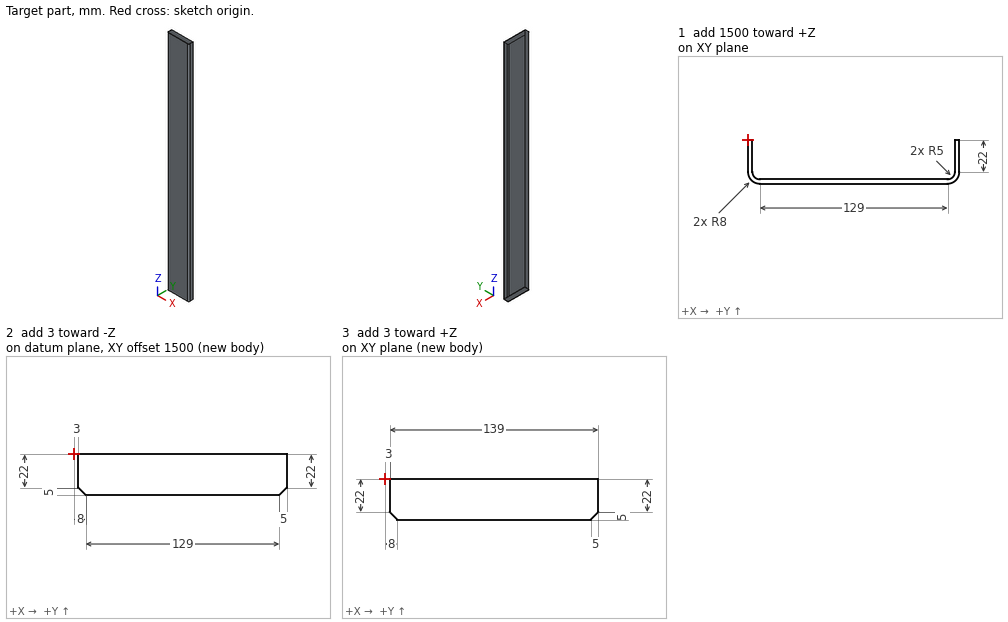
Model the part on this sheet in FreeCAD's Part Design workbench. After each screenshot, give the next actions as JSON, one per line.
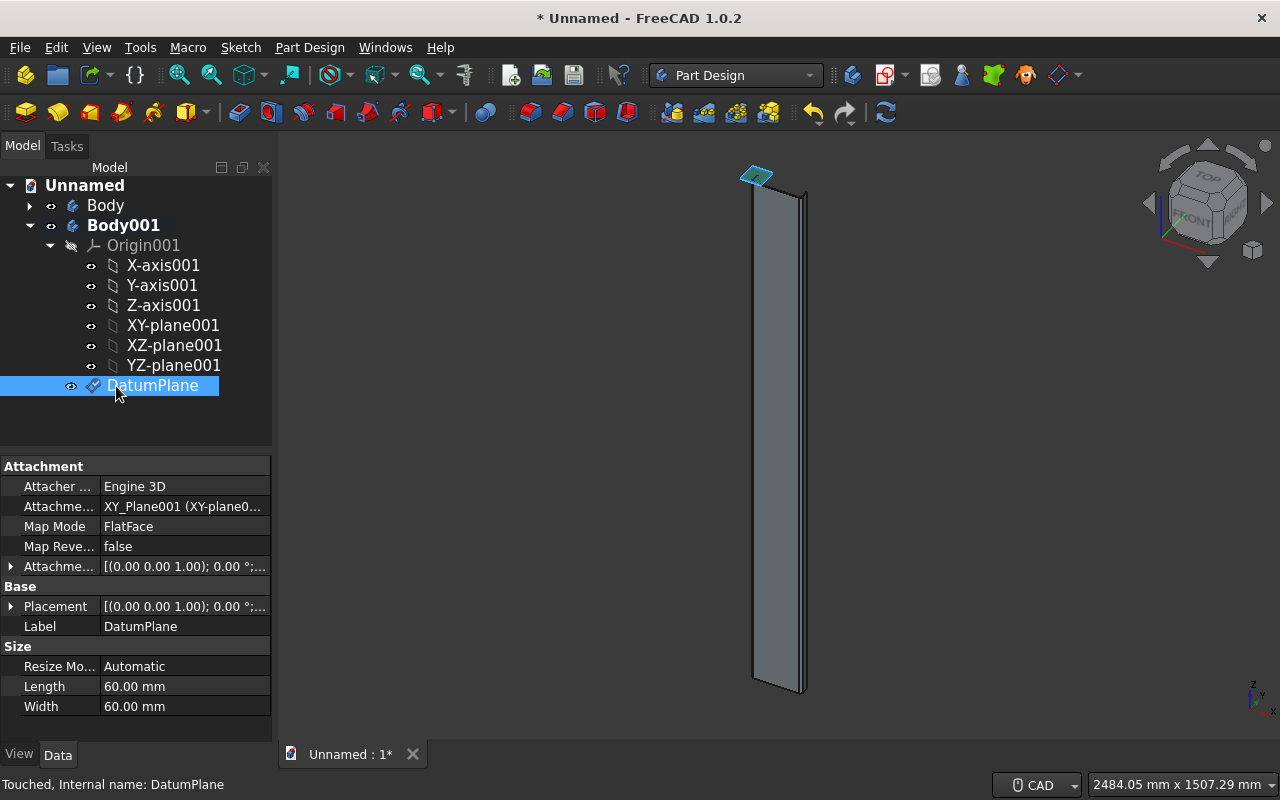
{"action": "left_click", "coordinate": [886, 76]}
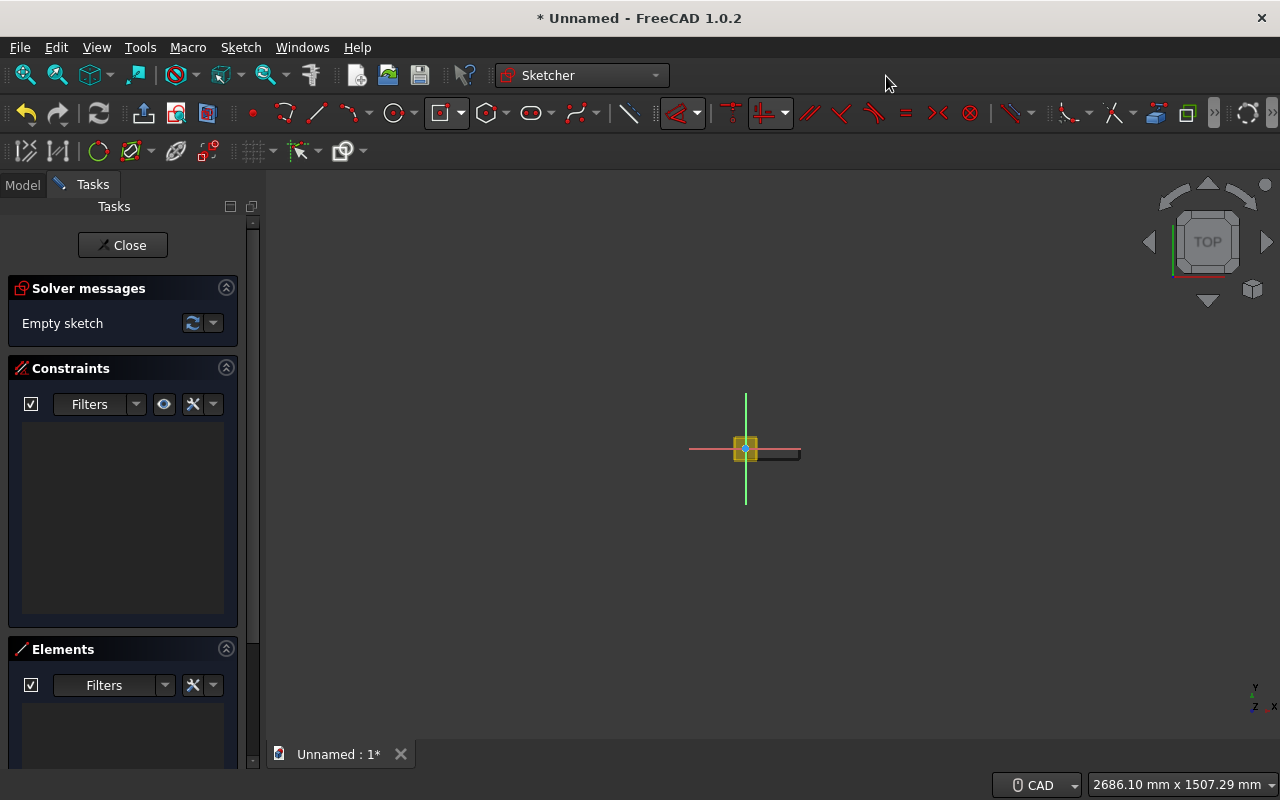
{"action": "scroll", "coordinate": [779, 454], "scroll_direction": "up", "scroll_amount": 12}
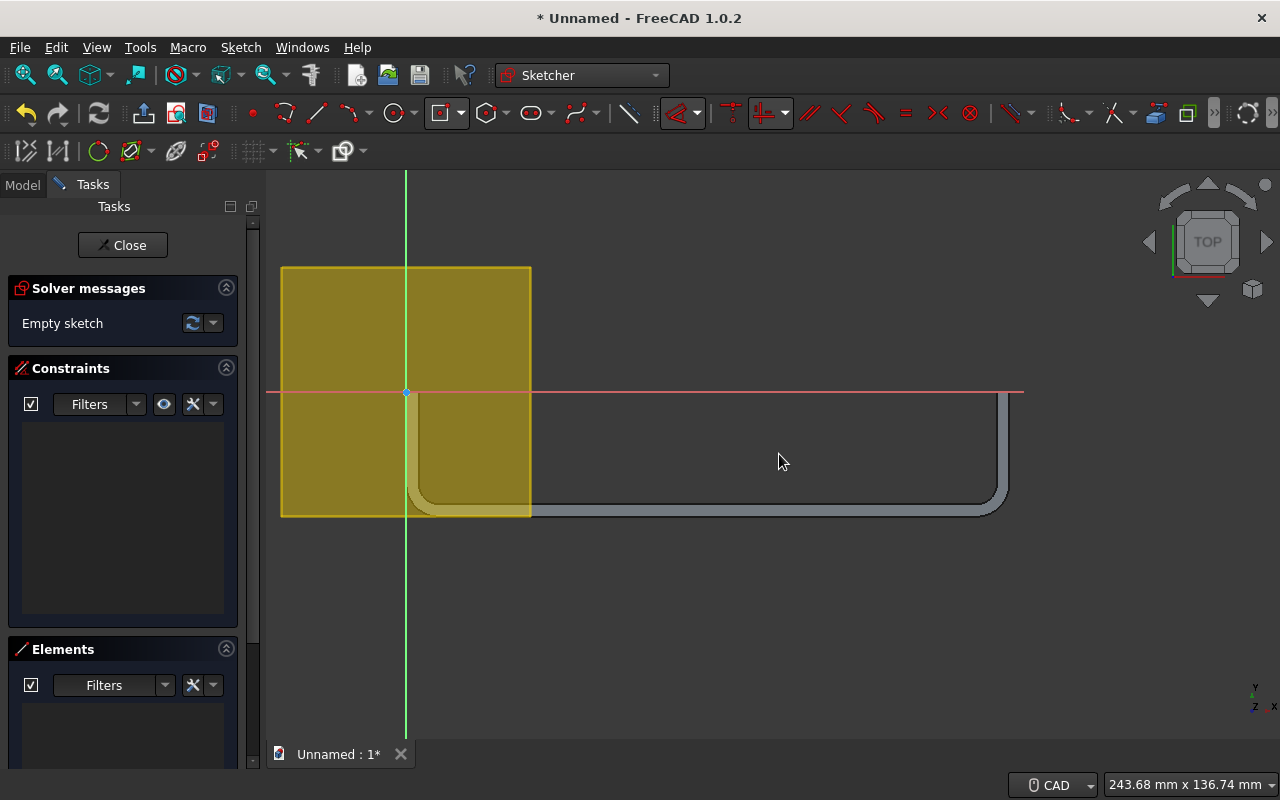
{"action": "key", "text": "g m"}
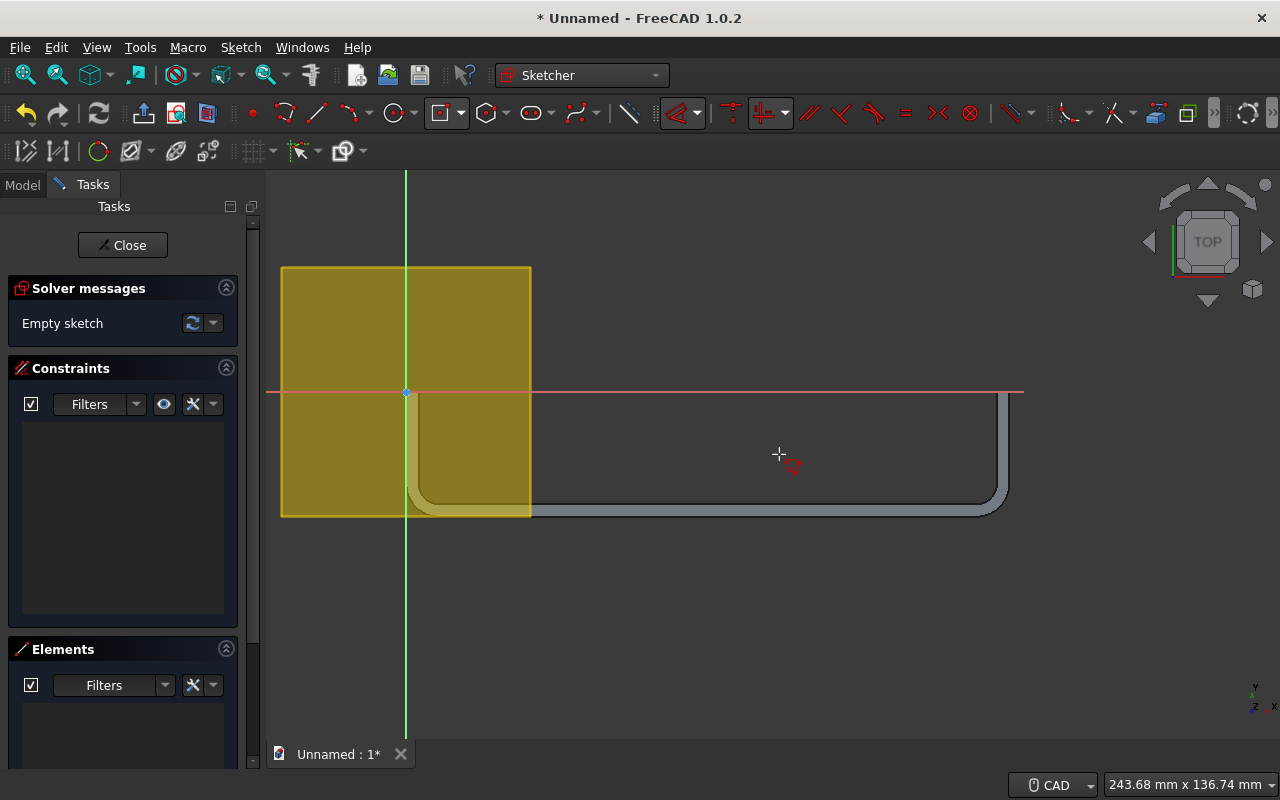
{"action": "scroll", "coordinate": [419, 392], "scroll_direction": "up", "scroll_amount": 2}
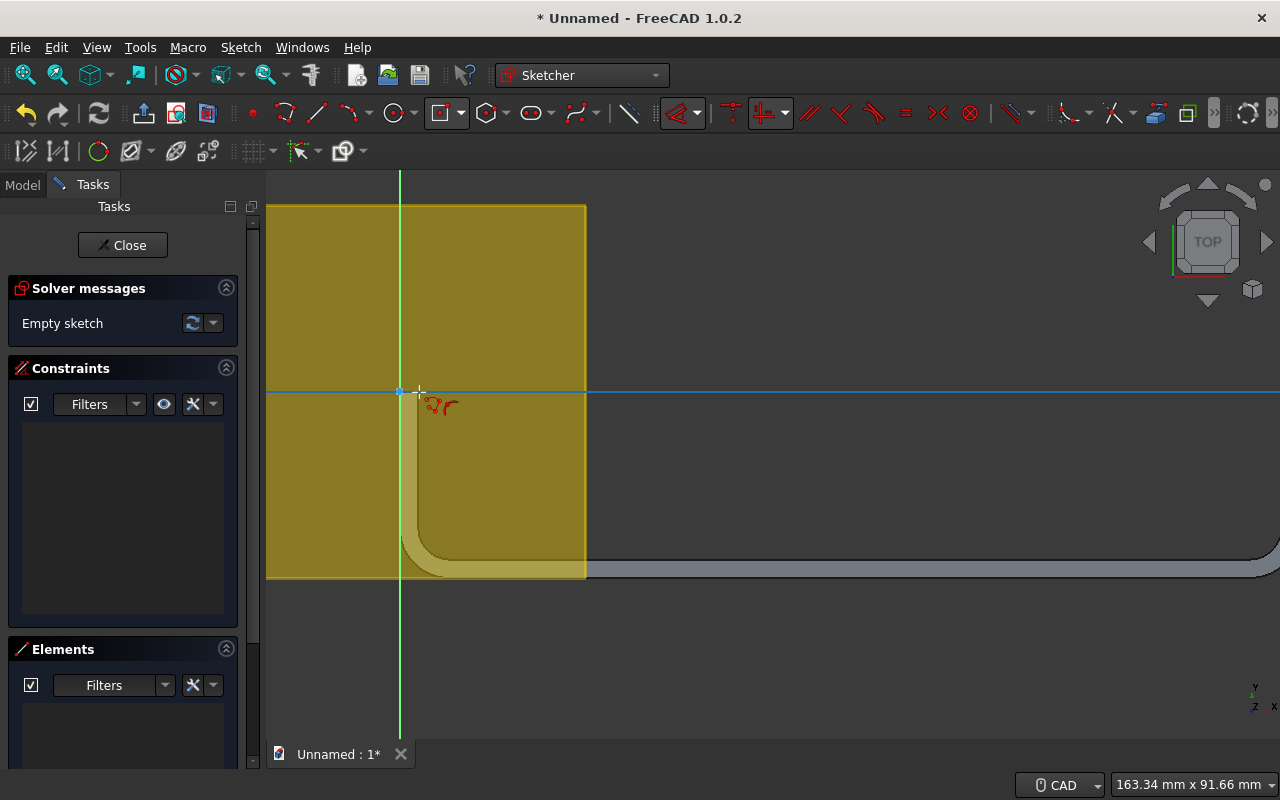
{"action": "left_click", "coordinate": [418, 392]}
{"action": "left_click", "coordinate": [418, 529]}
{"action": "left_click", "coordinate": [449, 560]}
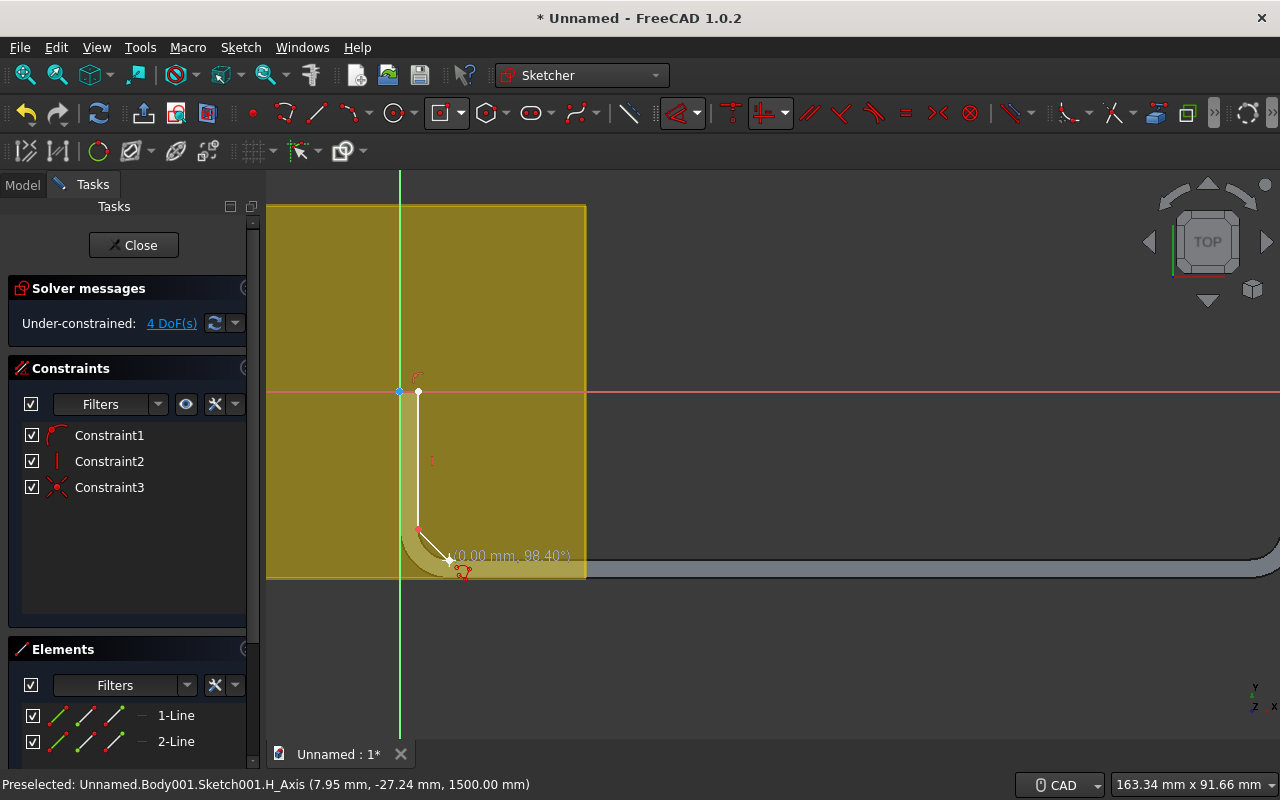
{"action": "scroll", "coordinate": [428, 411], "scroll_direction": "down", "scroll_amount": 2}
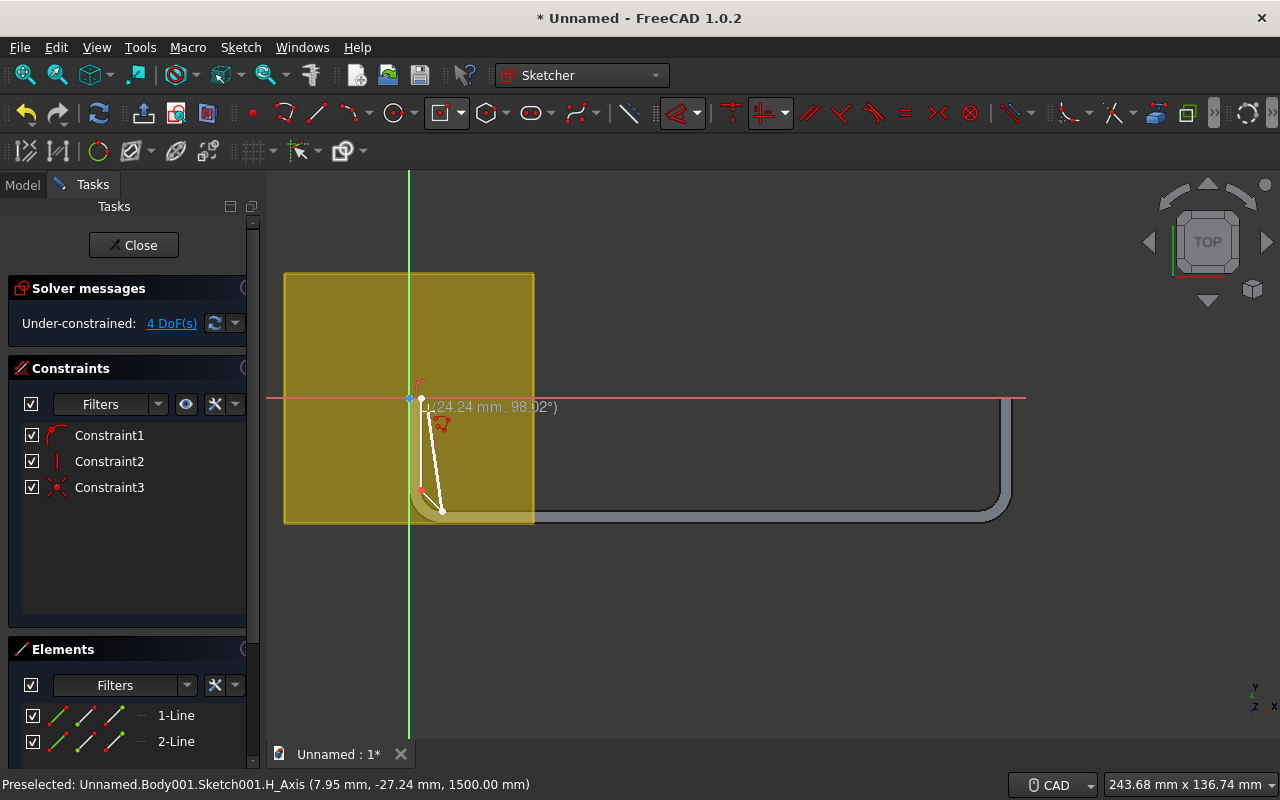
{"action": "left_click", "coordinate": [979, 511]}
{"action": "left_click", "coordinate": [1000, 490]}
{"action": "left_click", "coordinate": [1000, 407]}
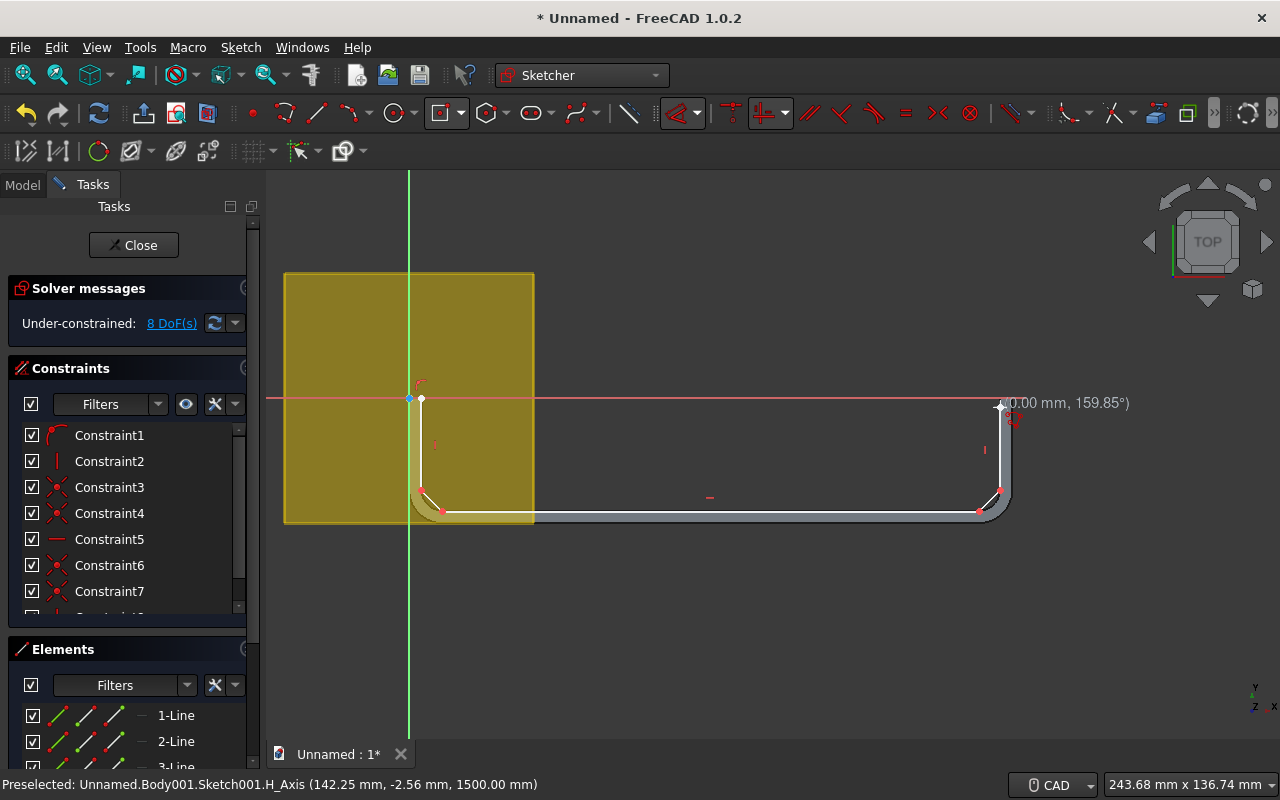
{"action": "scroll", "coordinate": [422, 398], "scroll_direction": "up", "scroll_amount": 2}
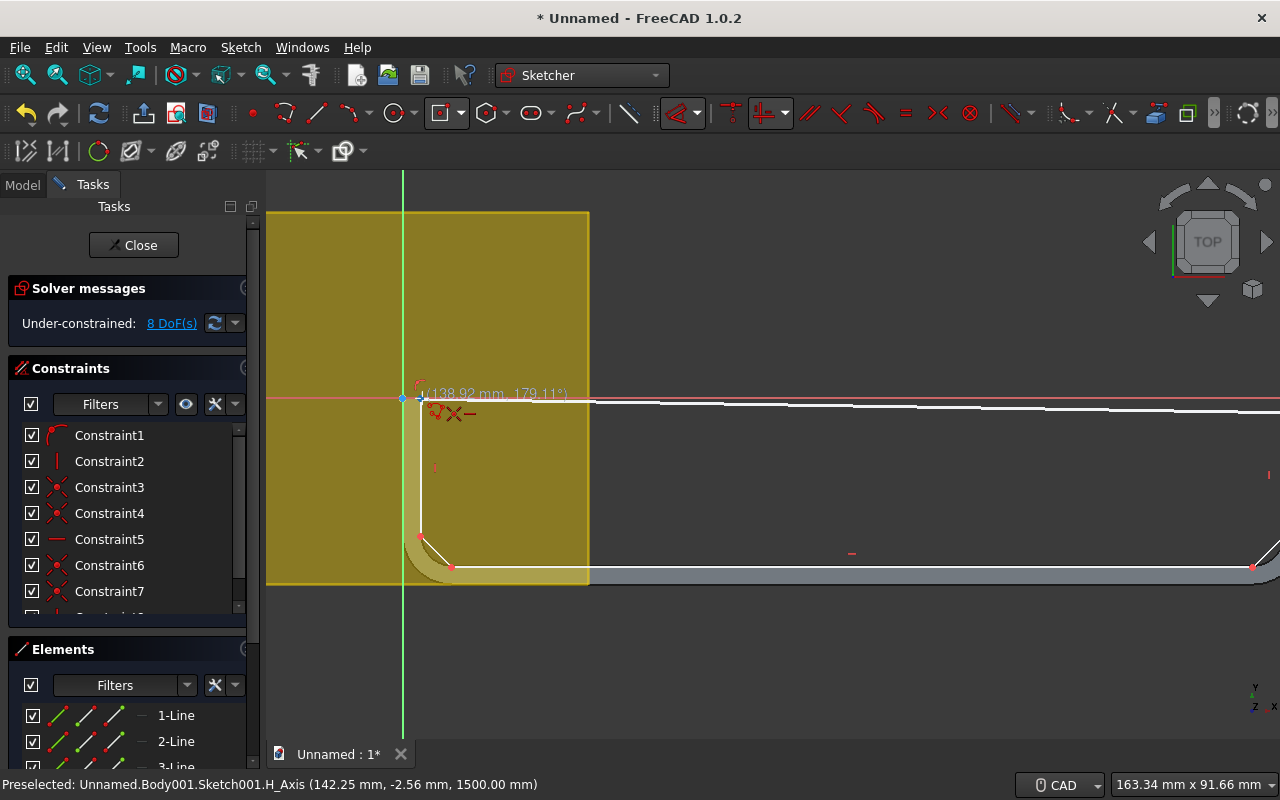
{"action": "left_click", "coordinate": [421, 398]}
{"action": "key", "text": "Escape"}
{"action": "key", "text": "Escape"}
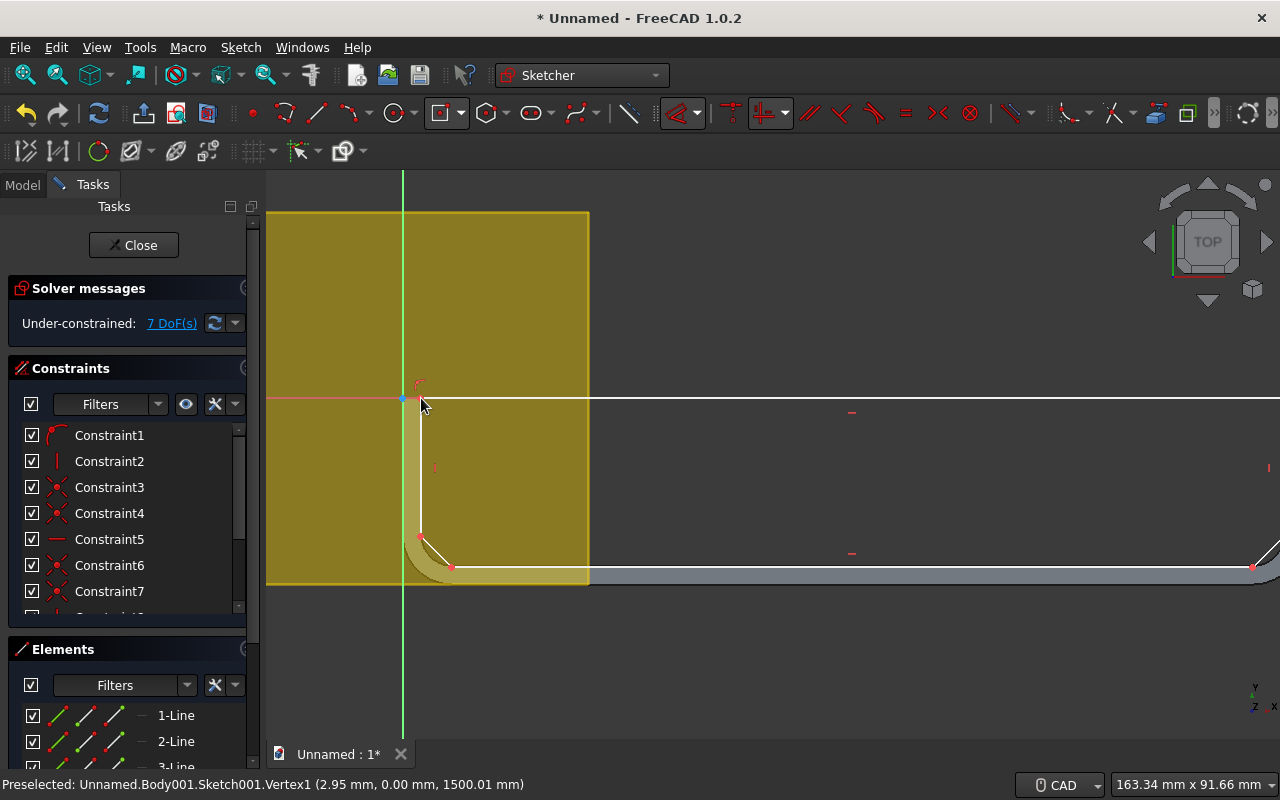
{"action": "left_click", "coordinate": [421, 440]}